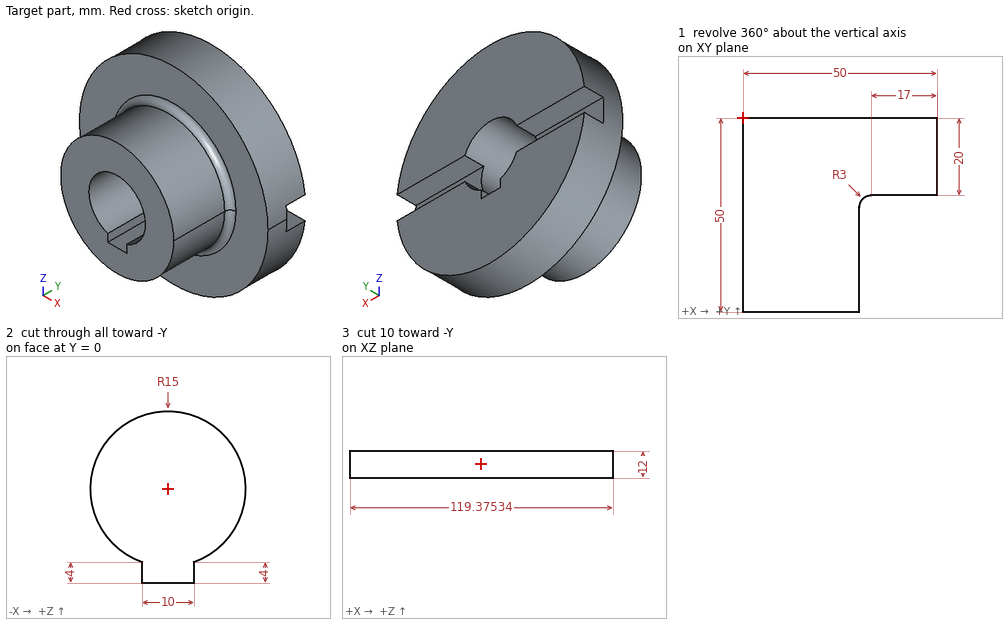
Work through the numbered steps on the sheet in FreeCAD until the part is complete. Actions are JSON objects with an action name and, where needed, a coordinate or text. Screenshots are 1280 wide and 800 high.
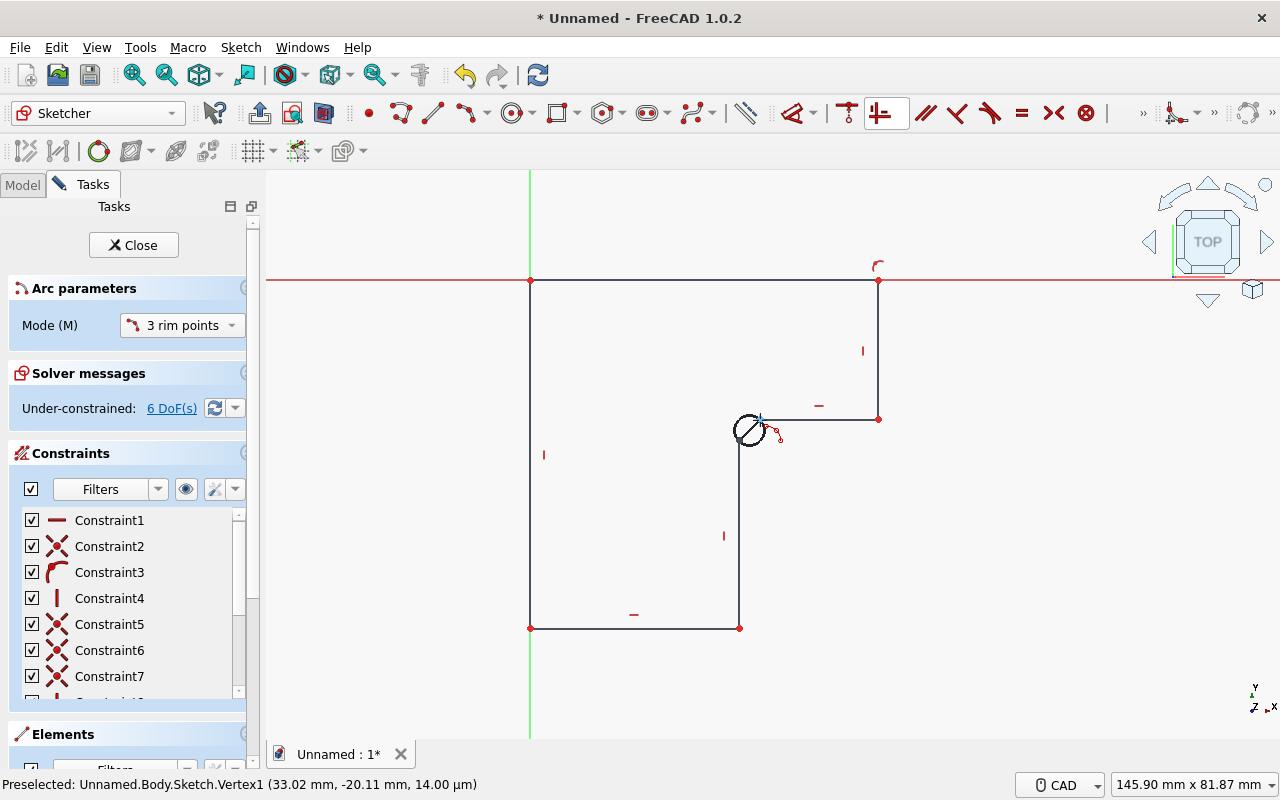
{"action": "scroll", "coordinate": [745, 425], "scroll_direction": "up", "scroll_amount": 5}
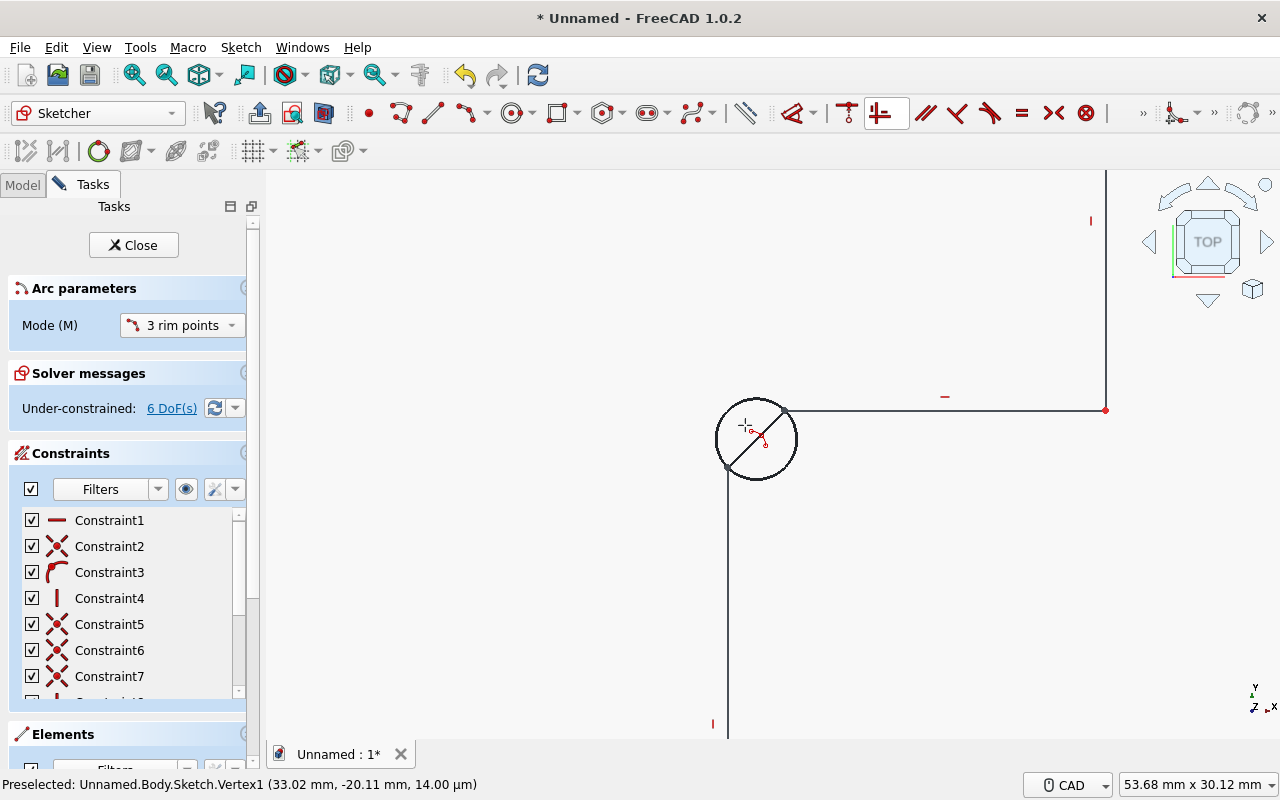
{"action": "left_click", "coordinate": [744, 425]}
{"action": "key", "text": "Escape"}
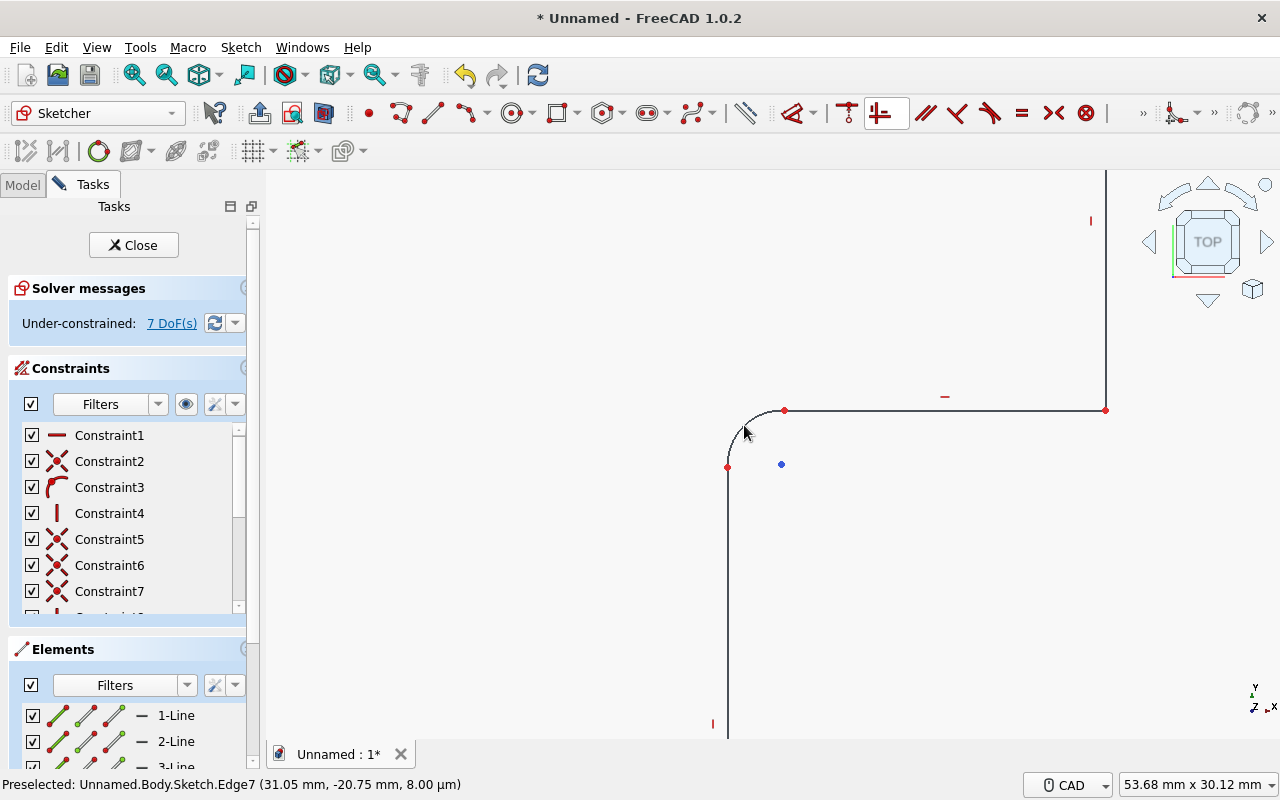
{"action": "left_click", "coordinate": [881, 411]}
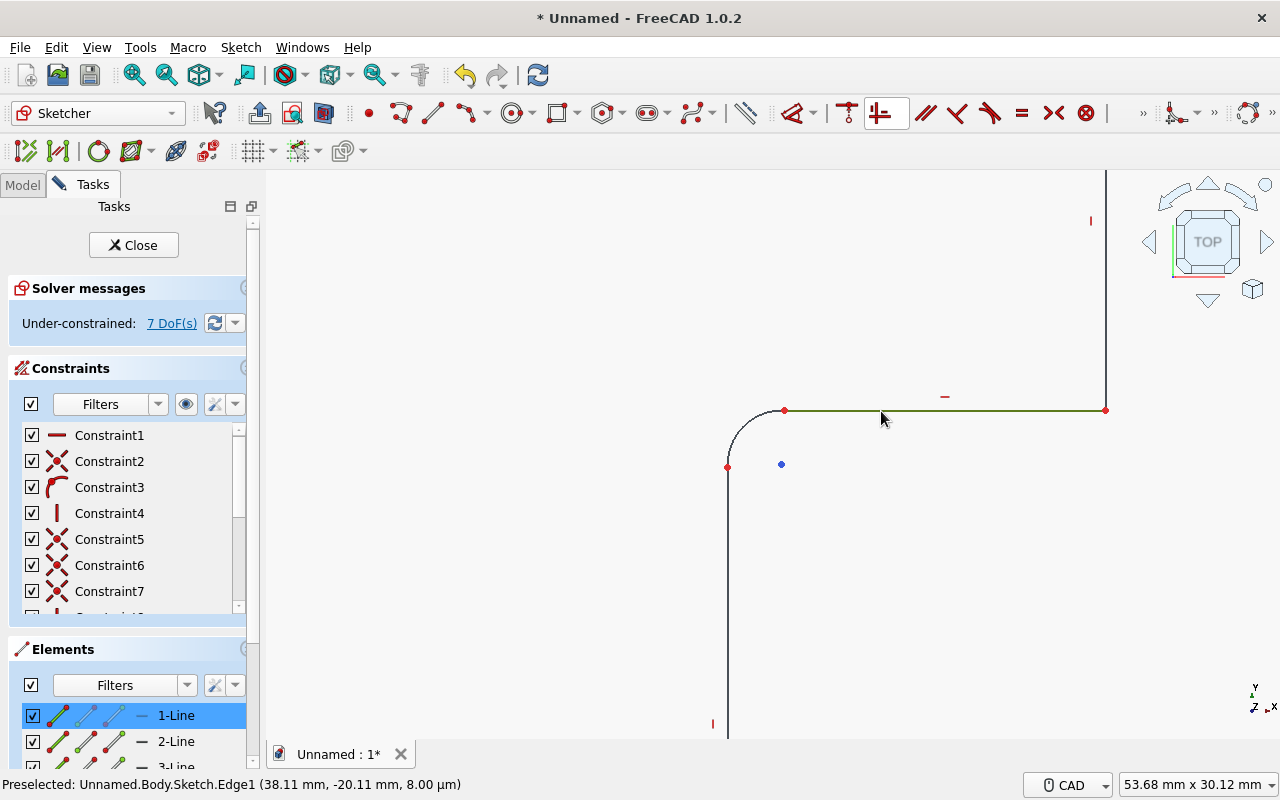
{"action": "left_click", "coordinate": [758, 416]}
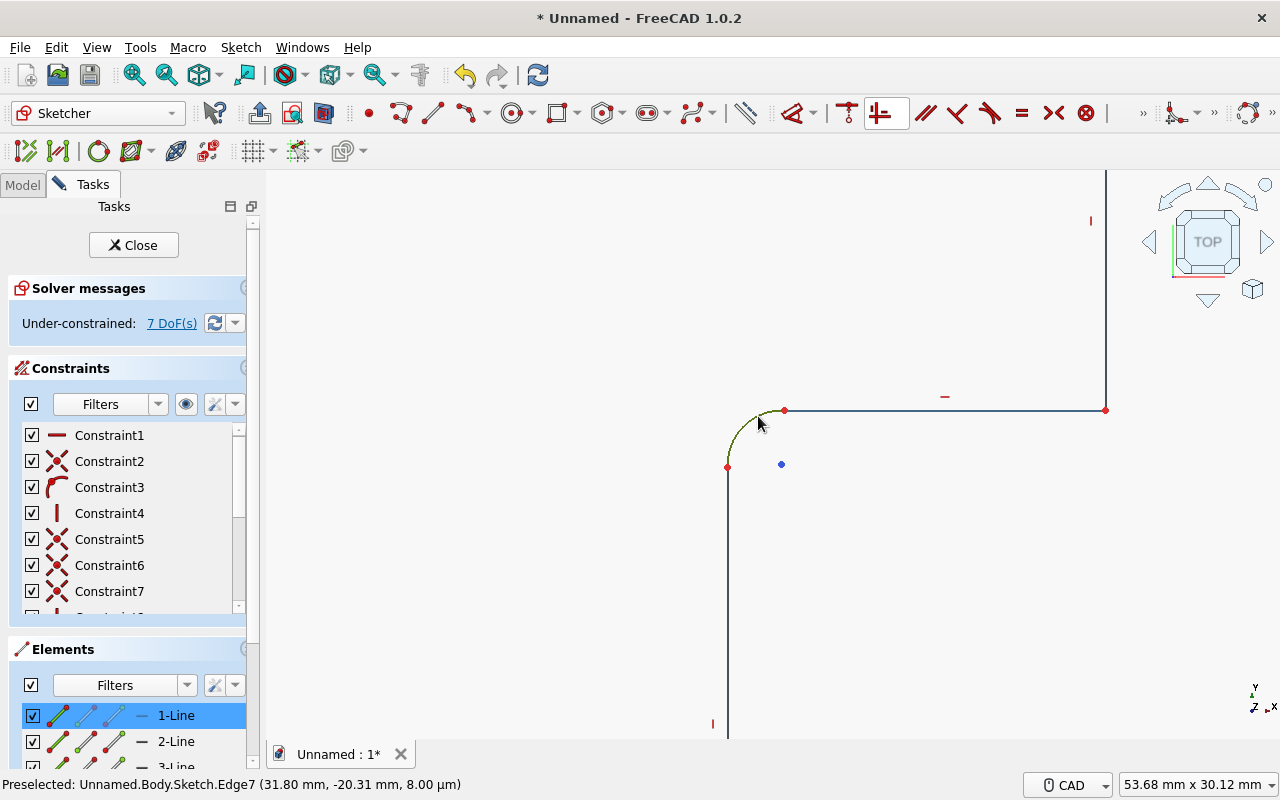
{"action": "left_click", "coordinate": [990, 114]}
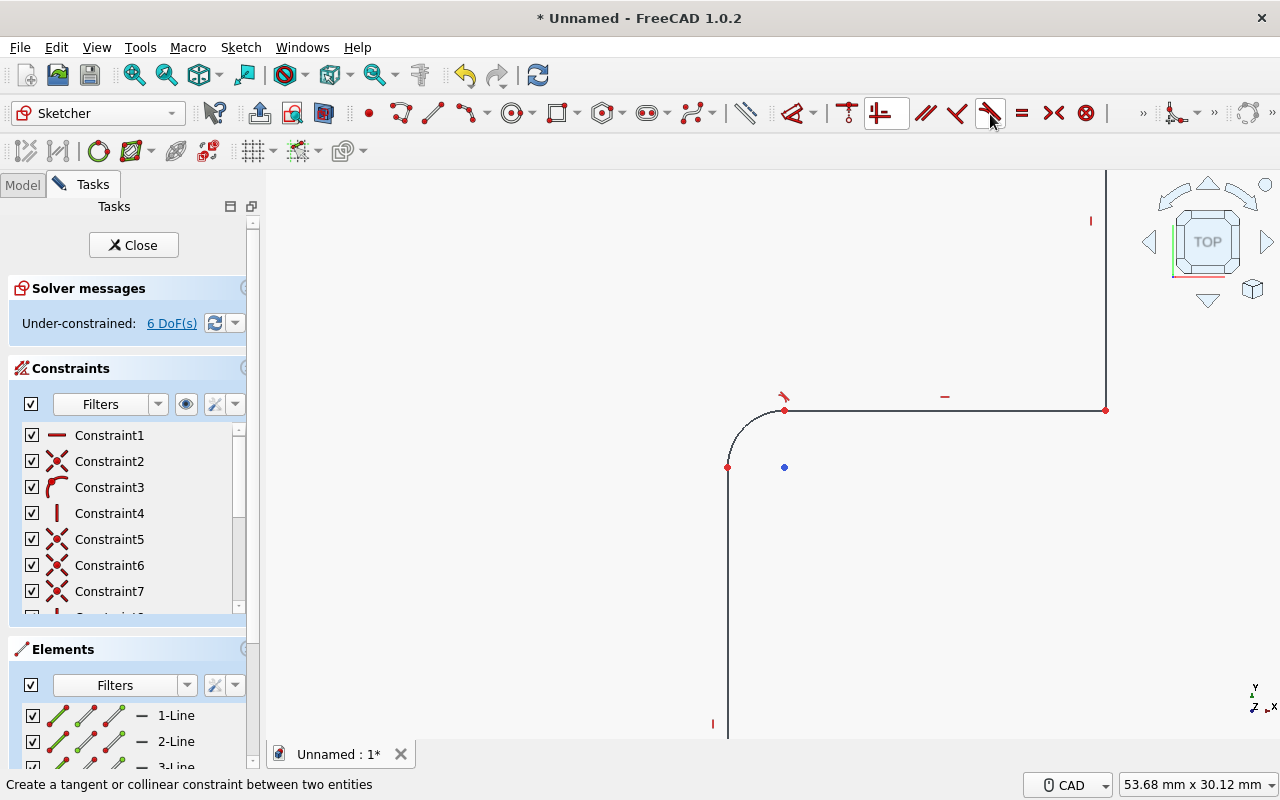
{"action": "left_click", "coordinate": [728, 621]}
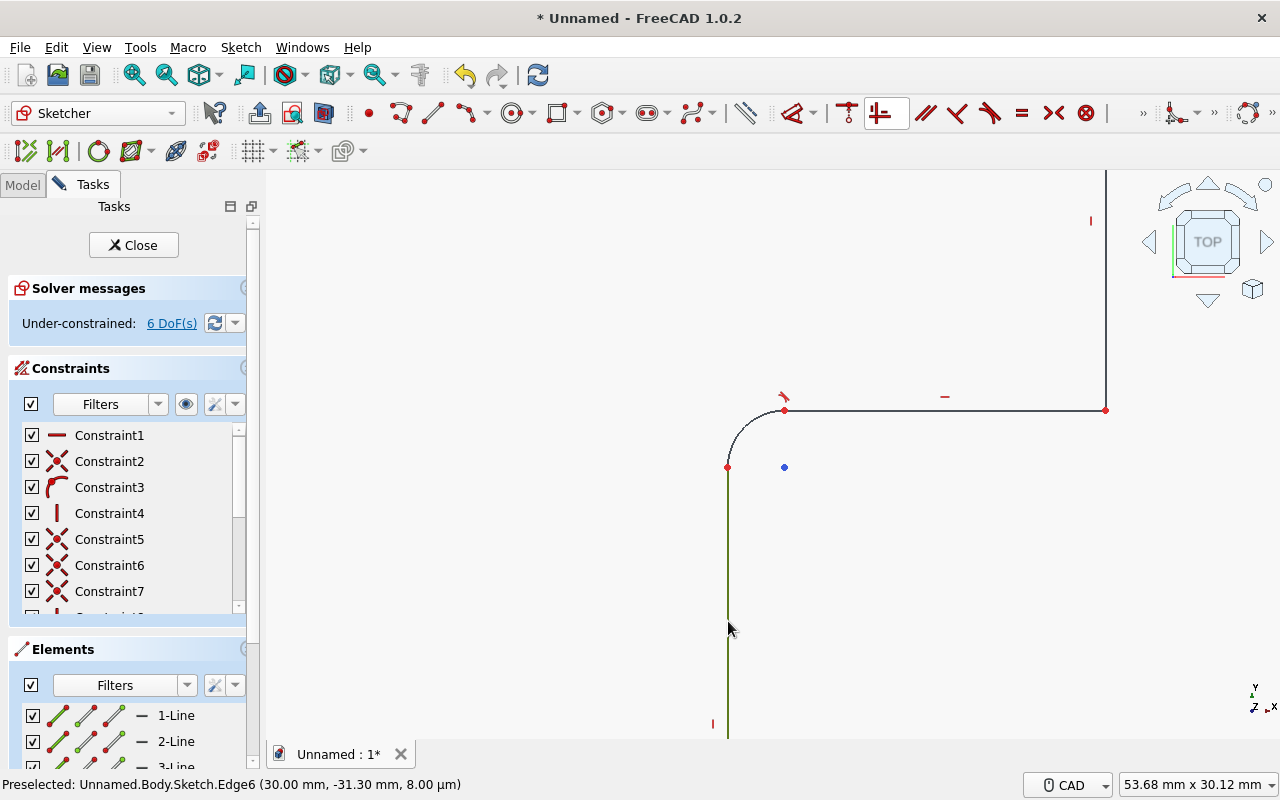
{"action": "left_click", "coordinate": [759, 417]}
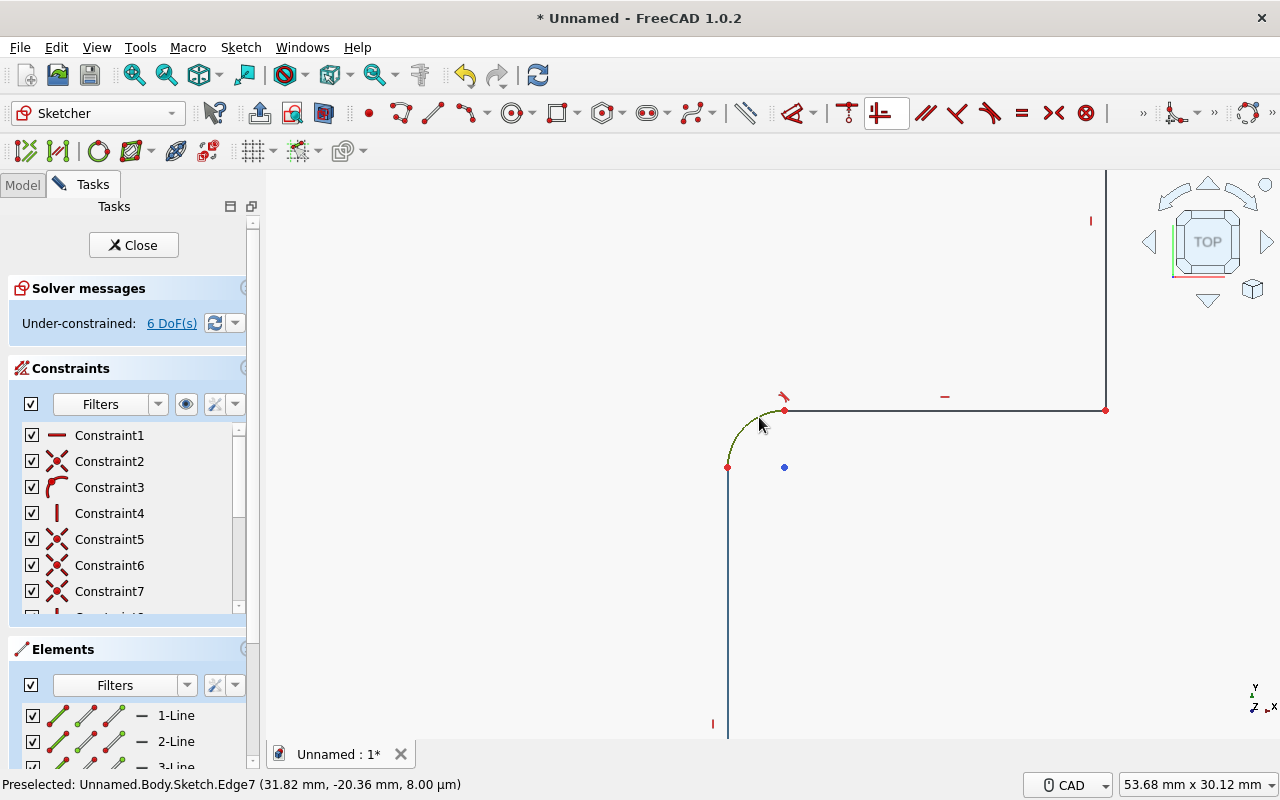
{"action": "left_click", "coordinate": [990, 114]}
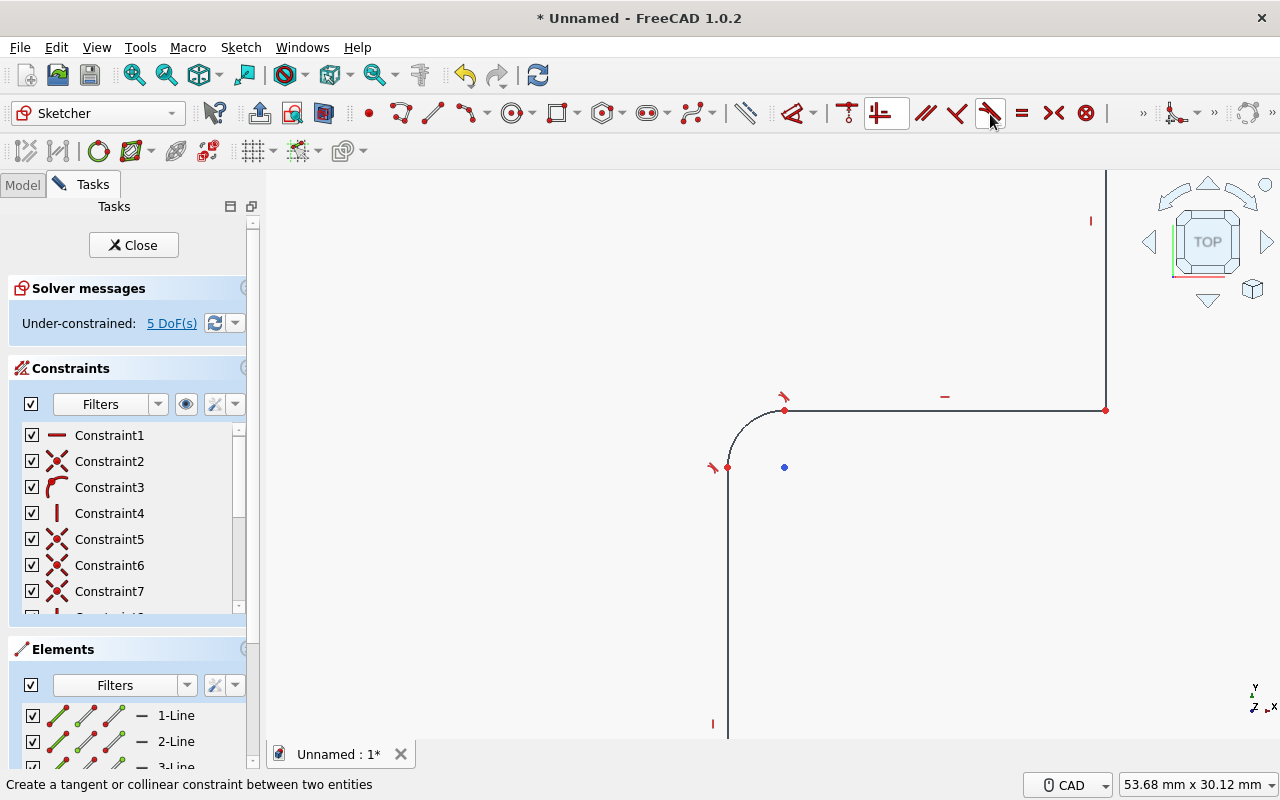
{"action": "left_click", "coordinate": [792, 114]}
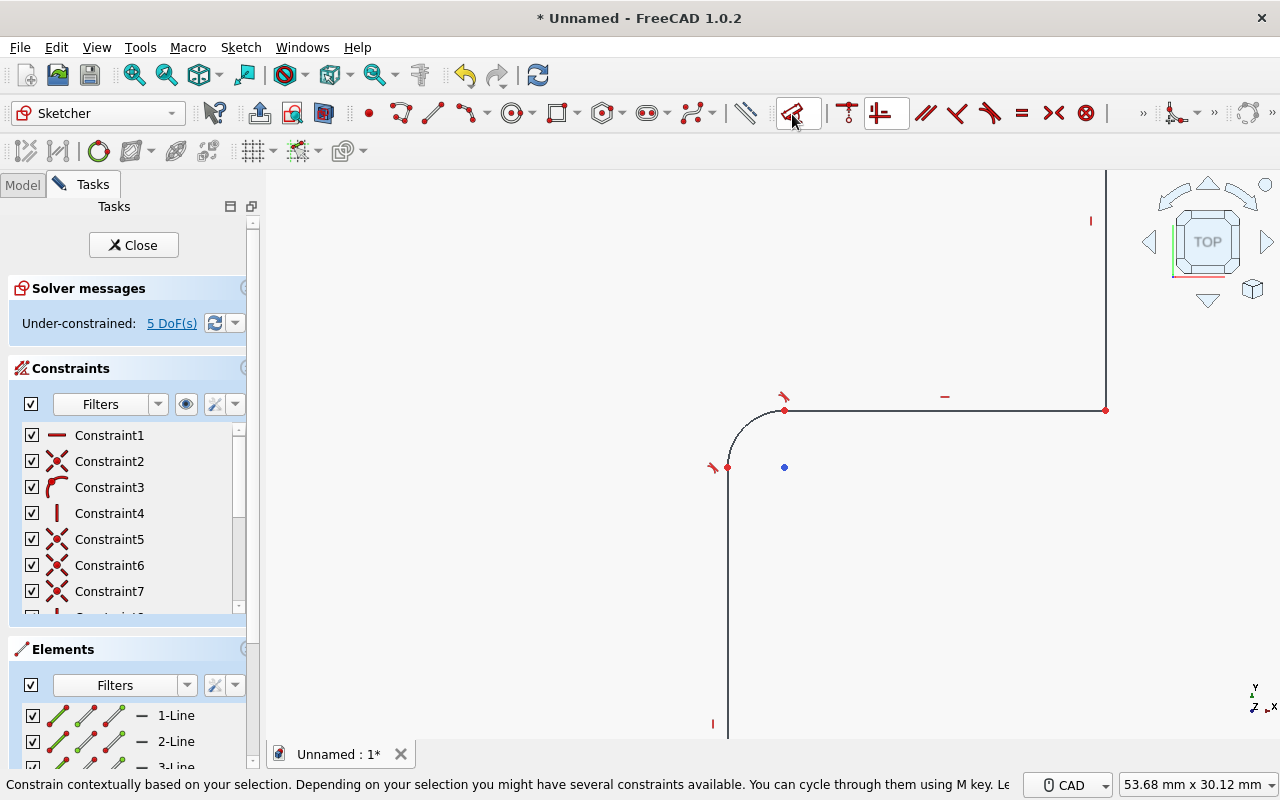
{"action": "left_click", "coordinate": [759, 417]}
{"action": "left_click", "coordinate": [744, 388]}